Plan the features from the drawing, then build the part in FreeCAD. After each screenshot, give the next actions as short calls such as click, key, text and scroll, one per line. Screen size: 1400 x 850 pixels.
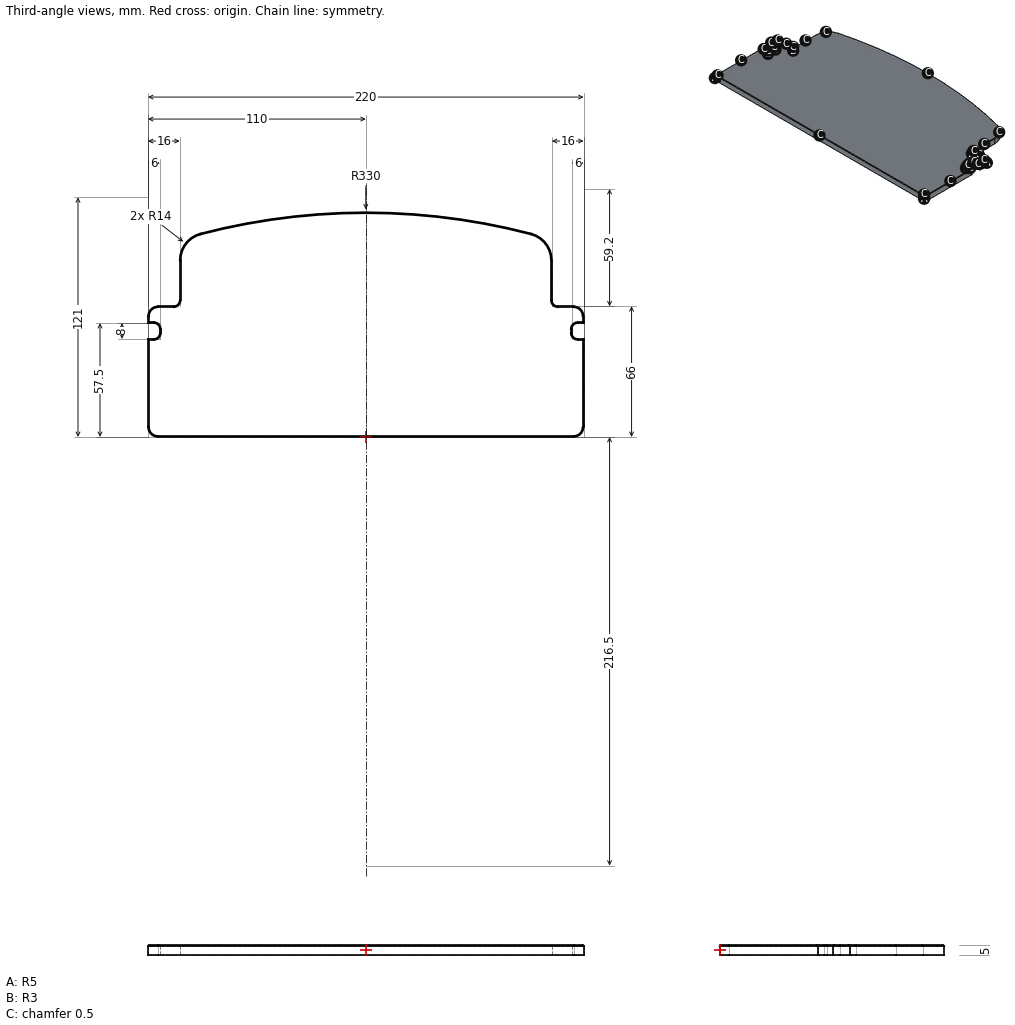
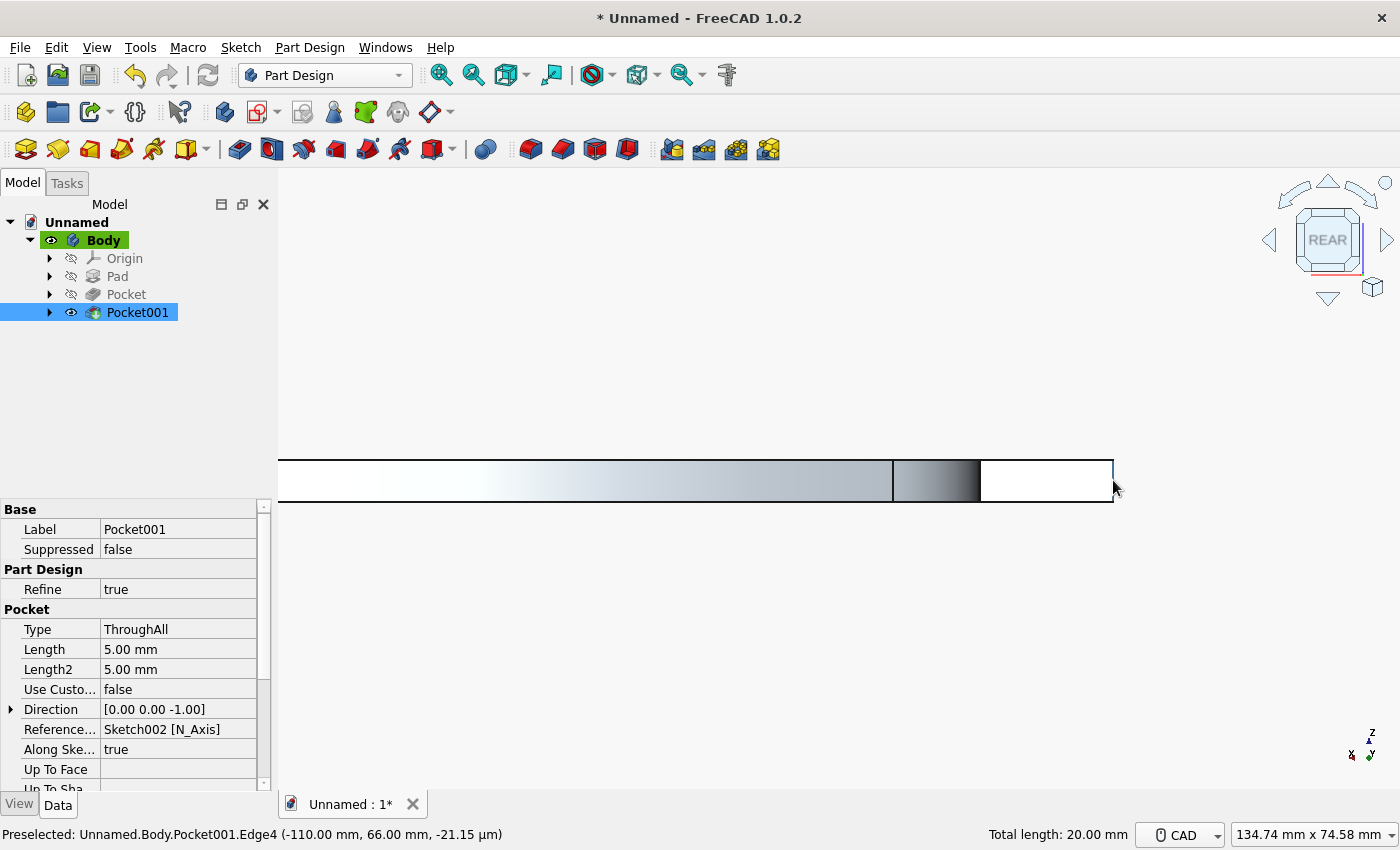
click(532, 150)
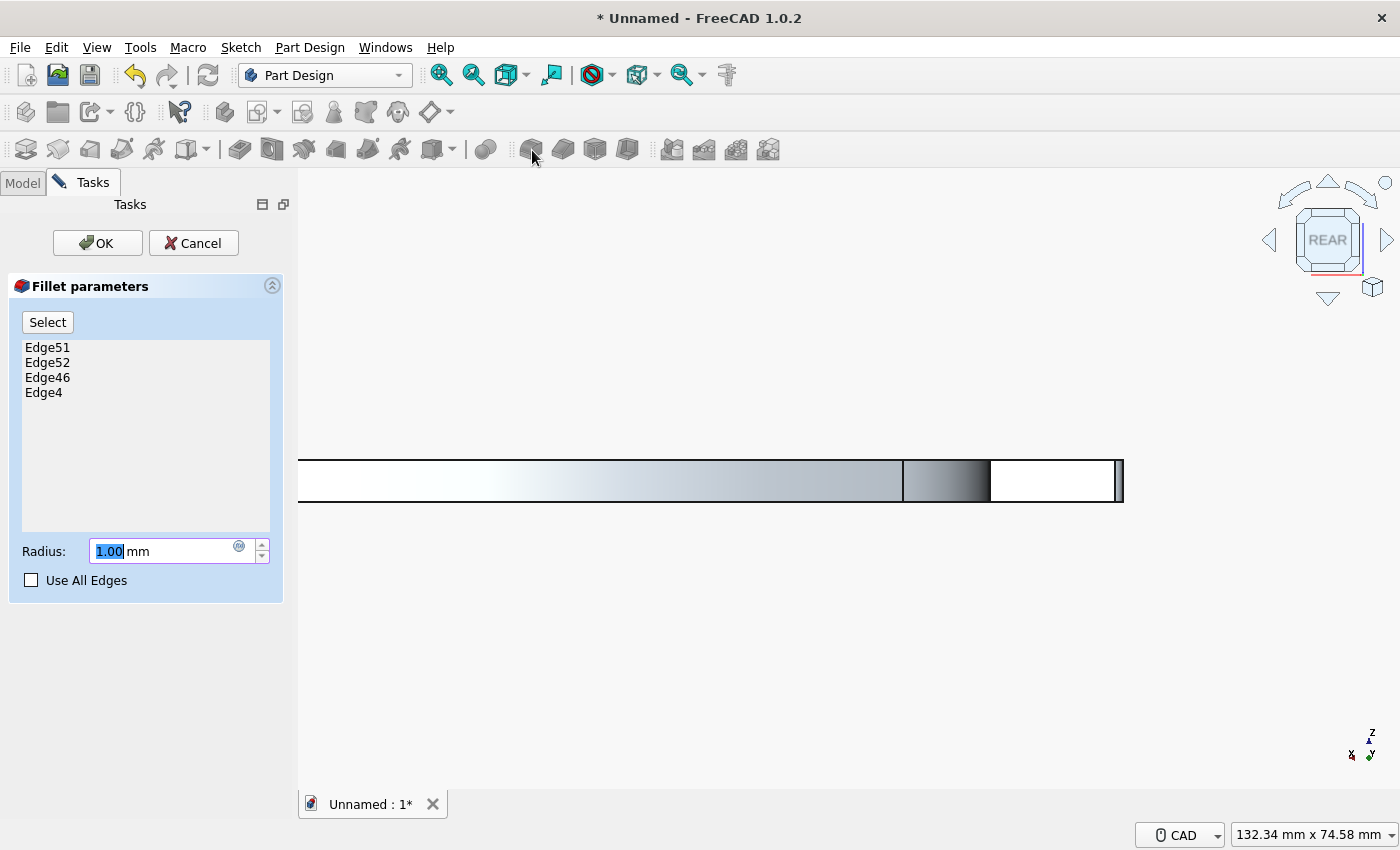
text(5)
key(Tab)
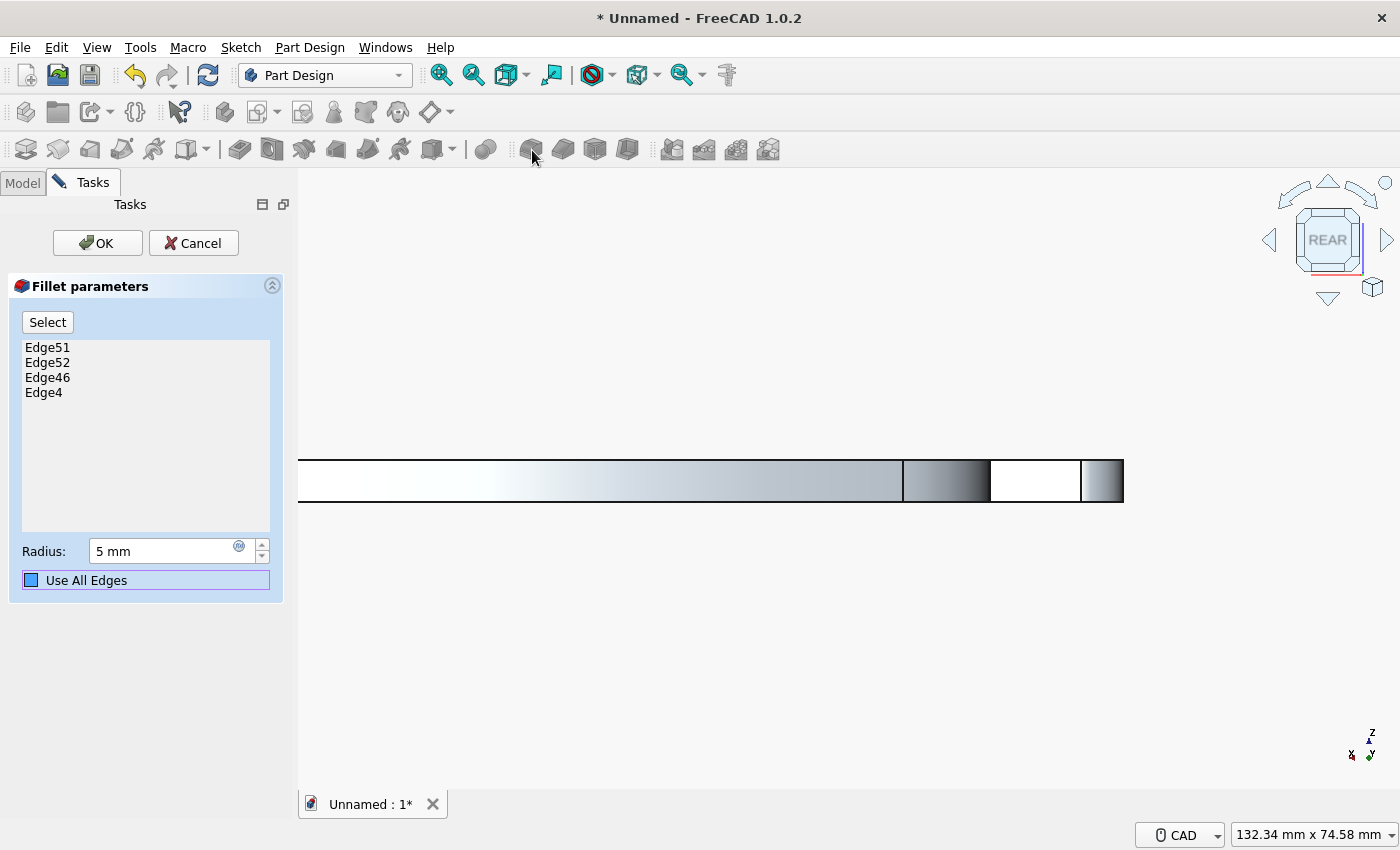
click(98, 243)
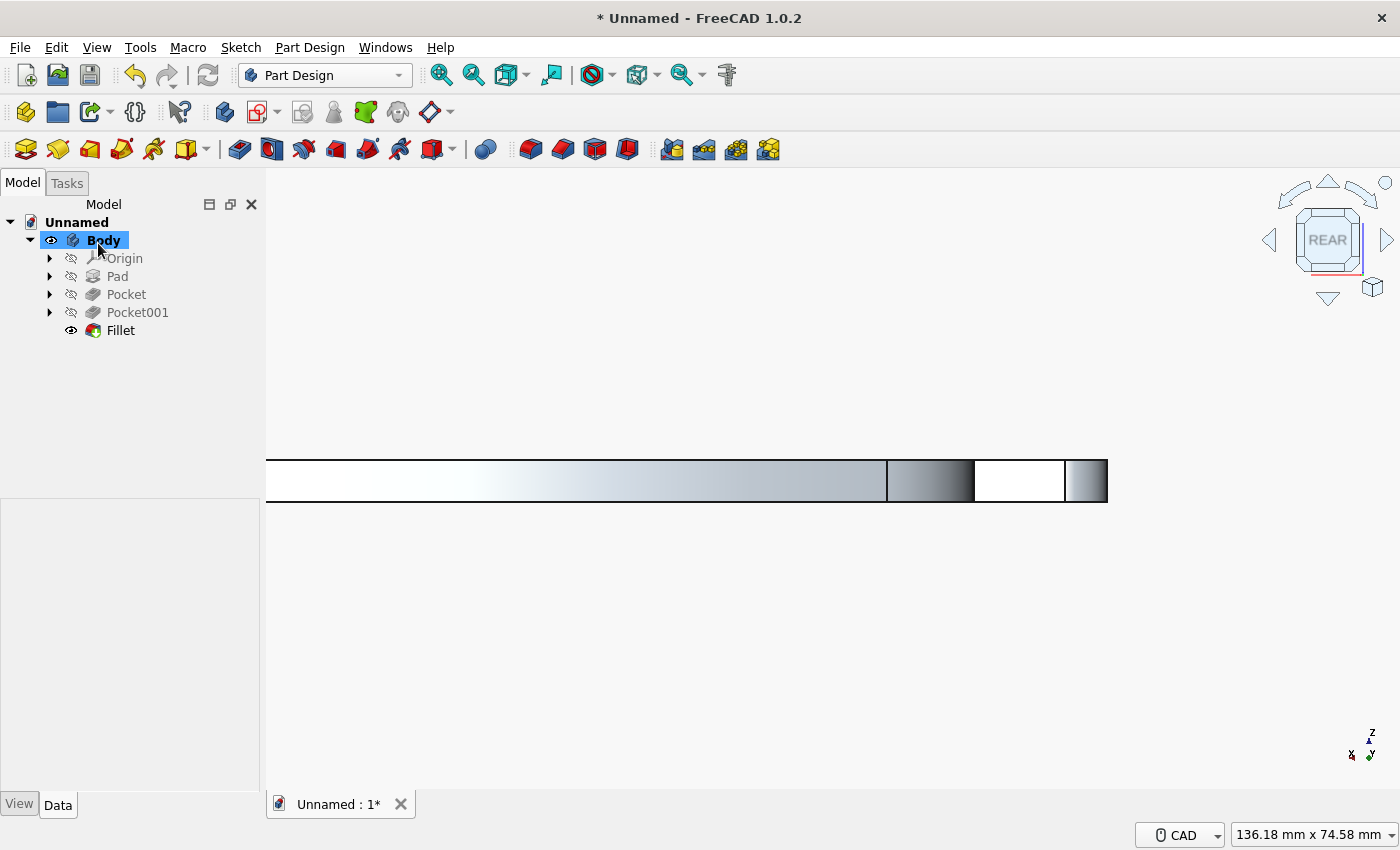
click(442, 76)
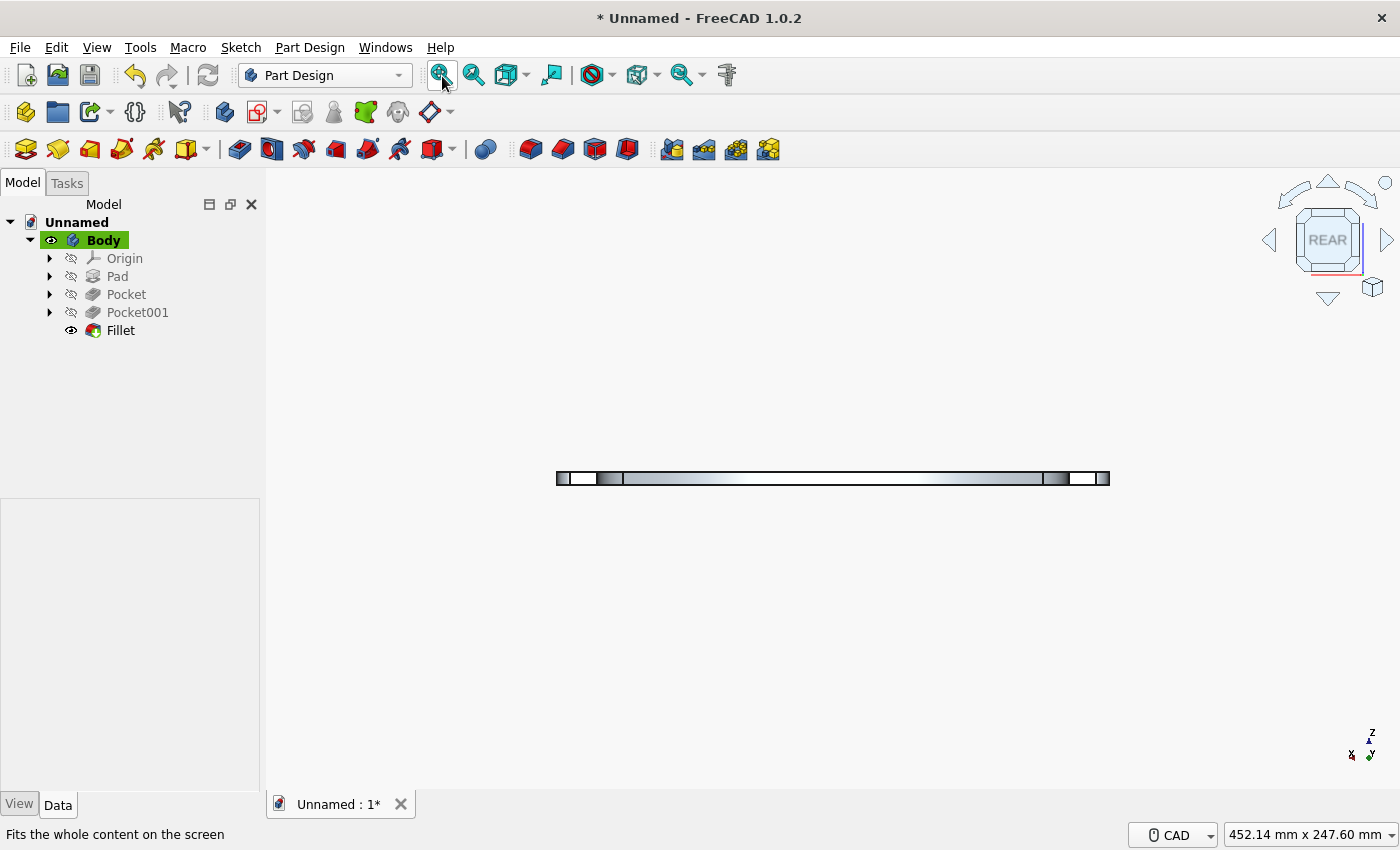
scroll(1069, 478, up, 6)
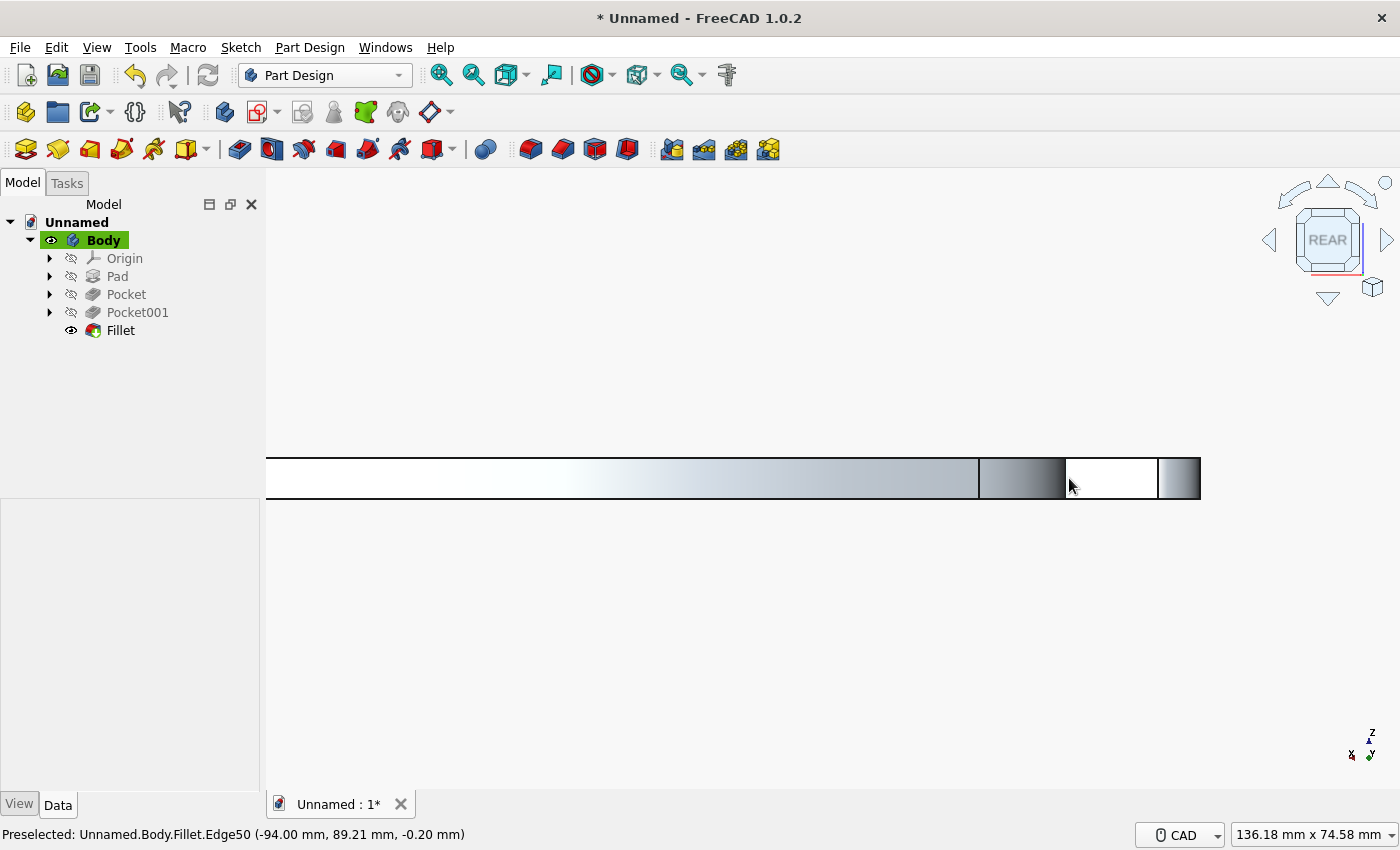
key(v)
key(f)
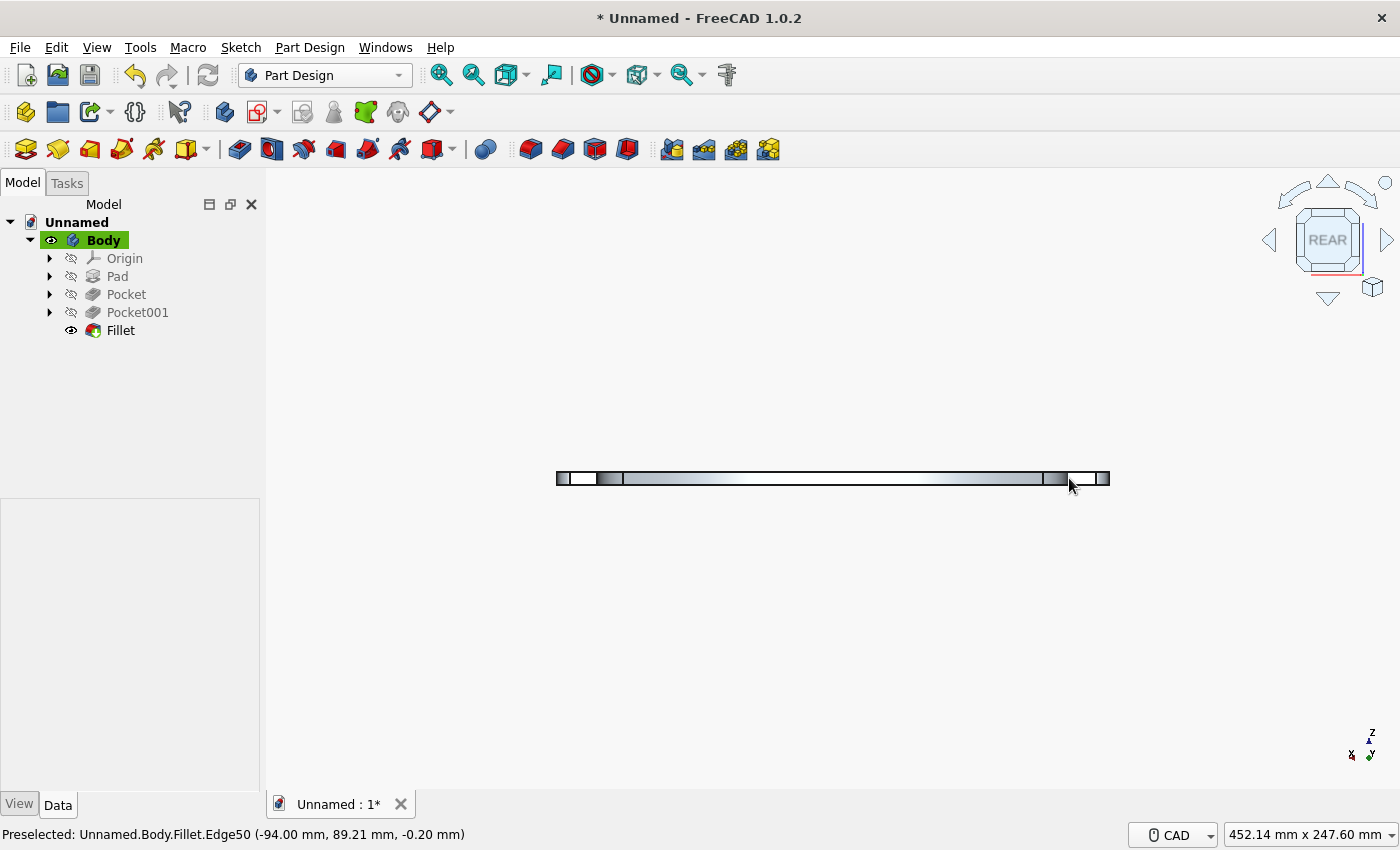
key(0)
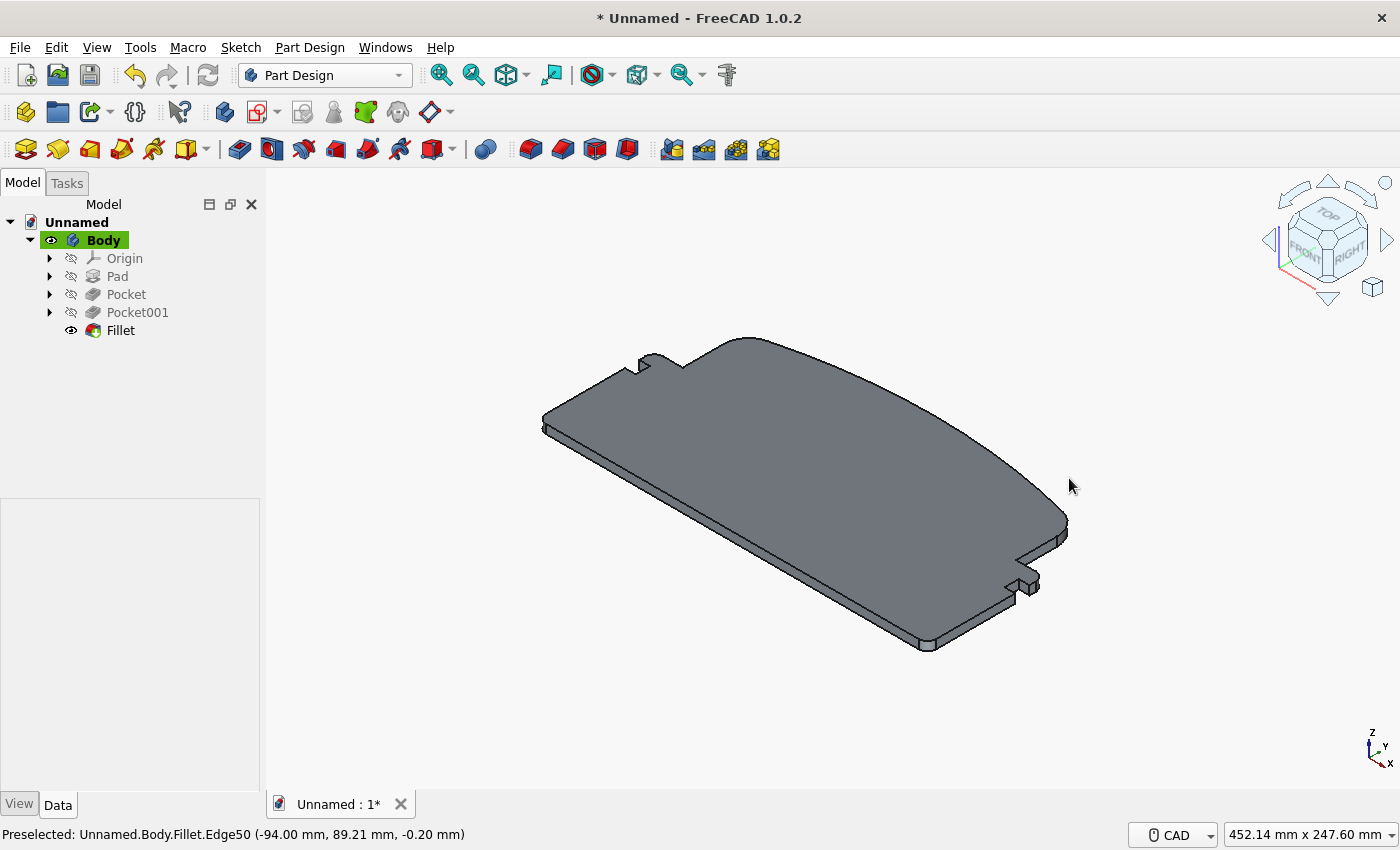
scroll(683, 372, up, 6)